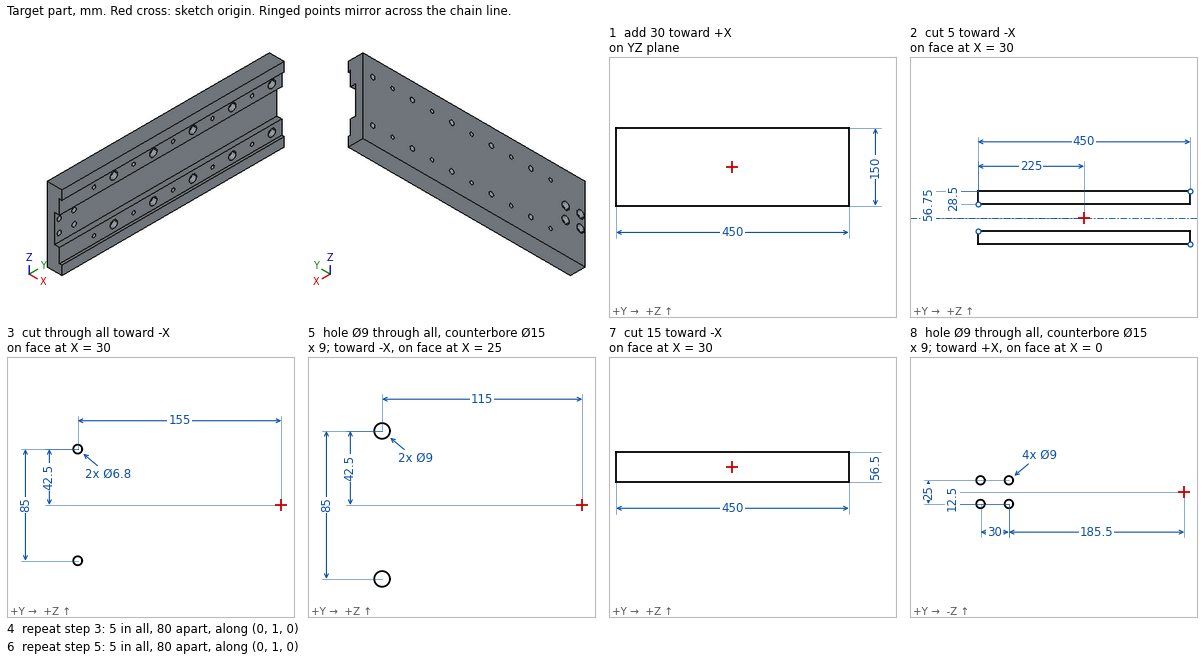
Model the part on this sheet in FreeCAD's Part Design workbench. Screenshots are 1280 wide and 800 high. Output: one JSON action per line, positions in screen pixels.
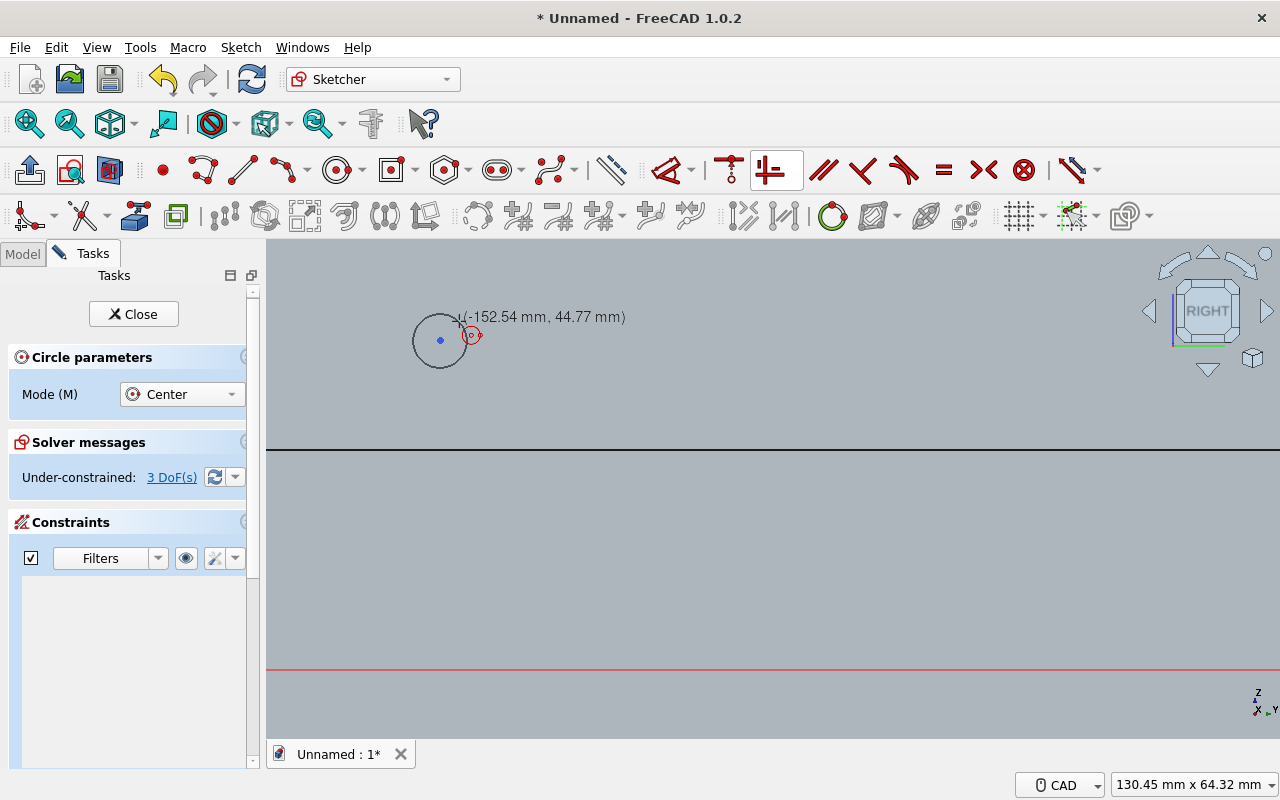
{"action": "scroll", "coordinate": [440, 341], "scroll_direction": "down", "scroll_amount": 4}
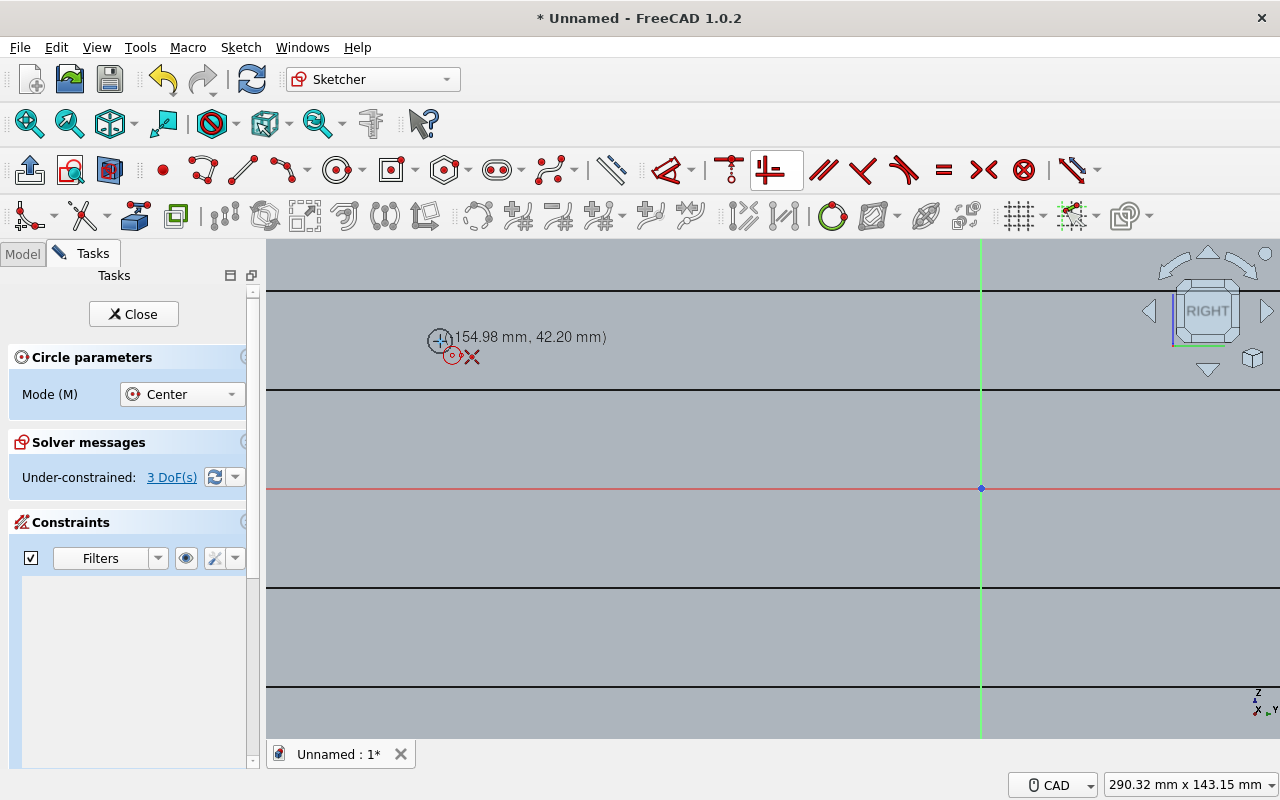
{"action": "scroll", "coordinate": [440, 637], "scroll_direction": "up", "scroll_amount": 4}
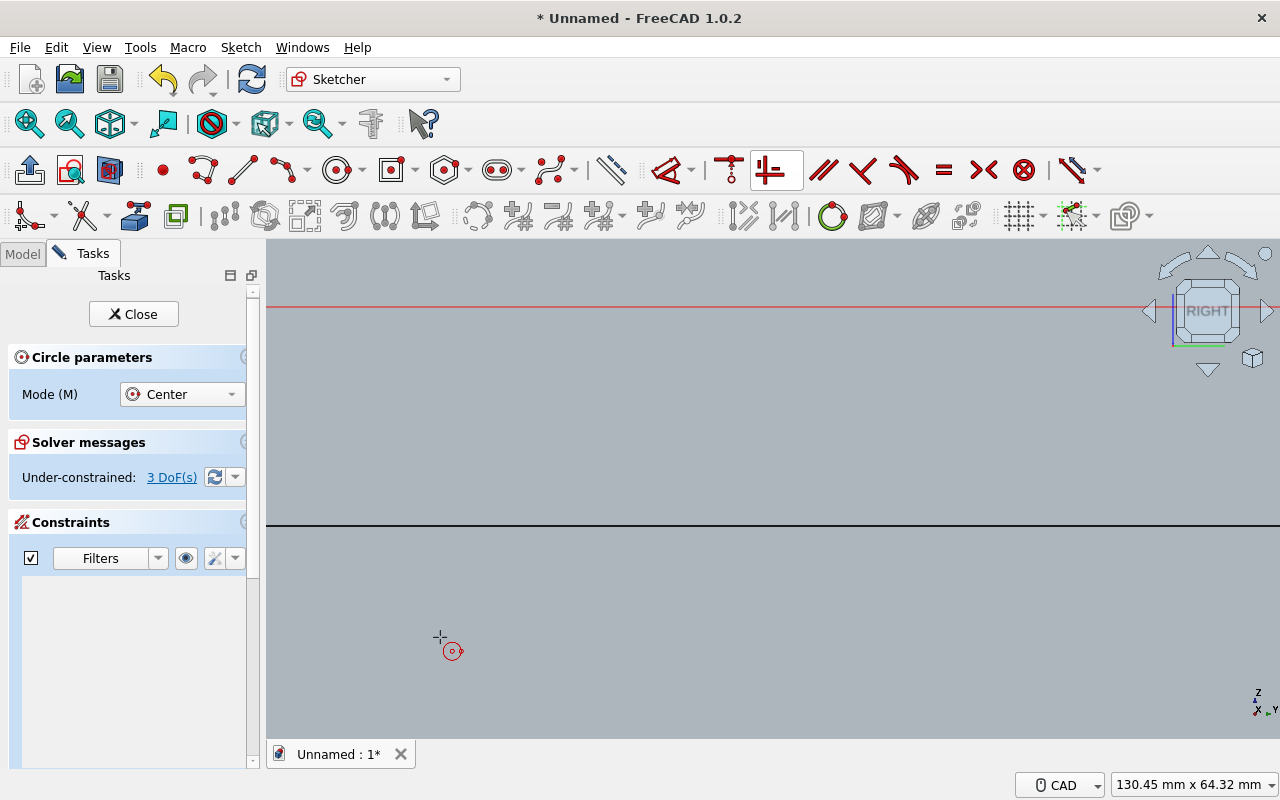
{"action": "left_click", "coordinate": [440, 637]}
{"action": "left_click", "coordinate": [459, 618]}
{"action": "key", "text": "Escape"}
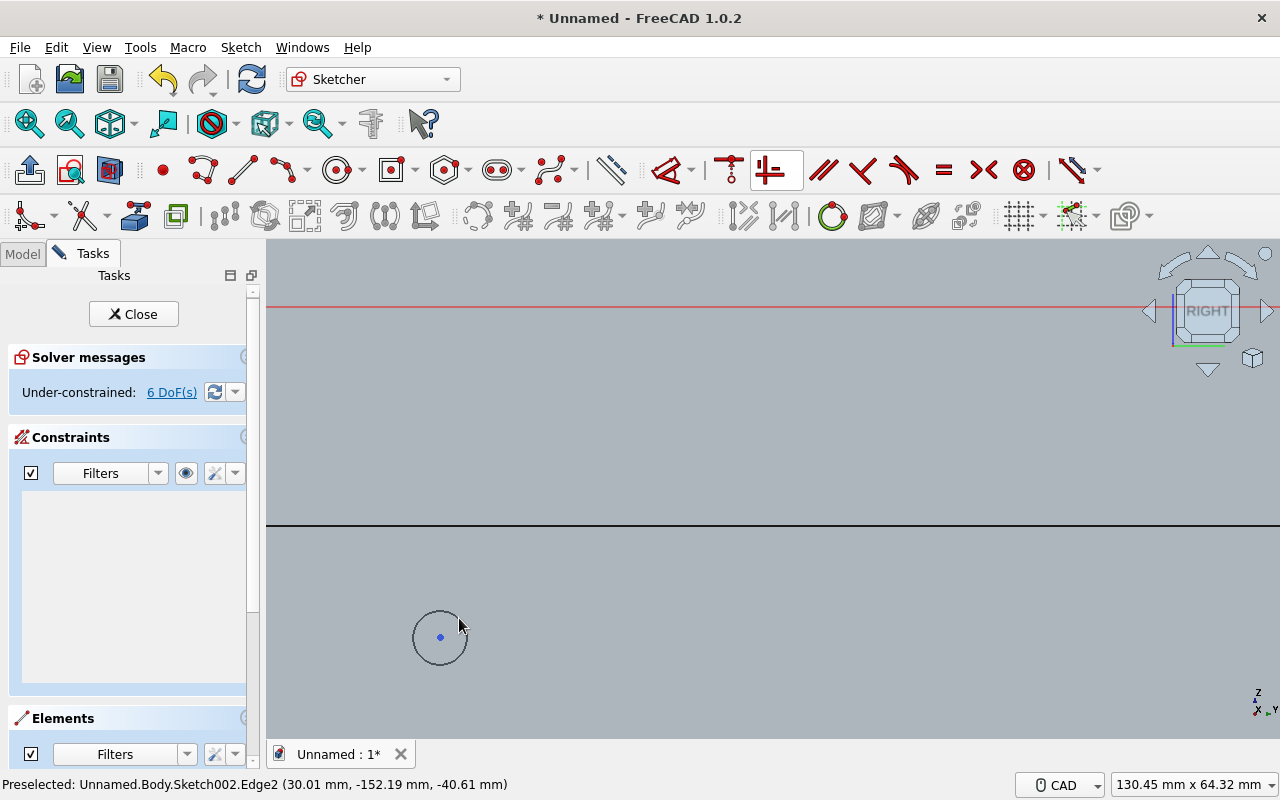
{"action": "scroll", "coordinate": [440, 638], "scroll_direction": "down", "scroll_amount": 4}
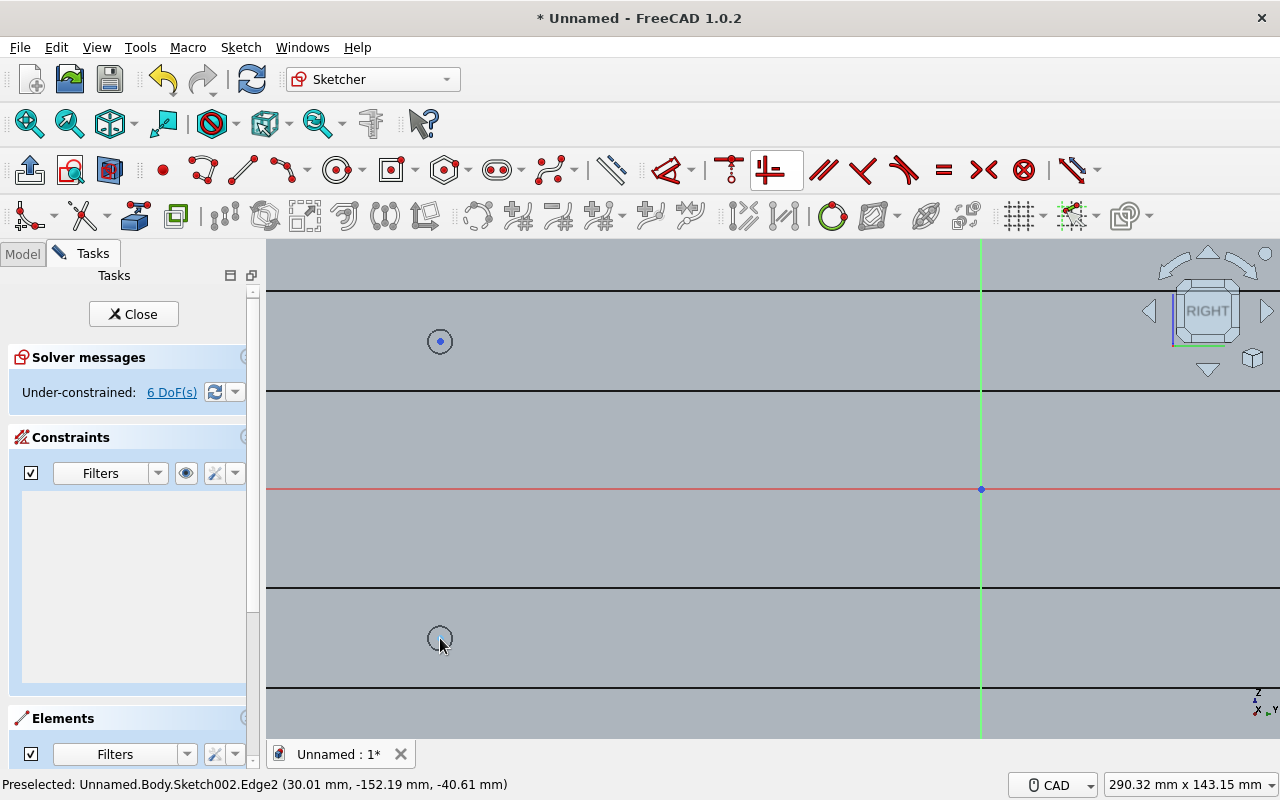
{"action": "left_click", "coordinate": [449, 333]}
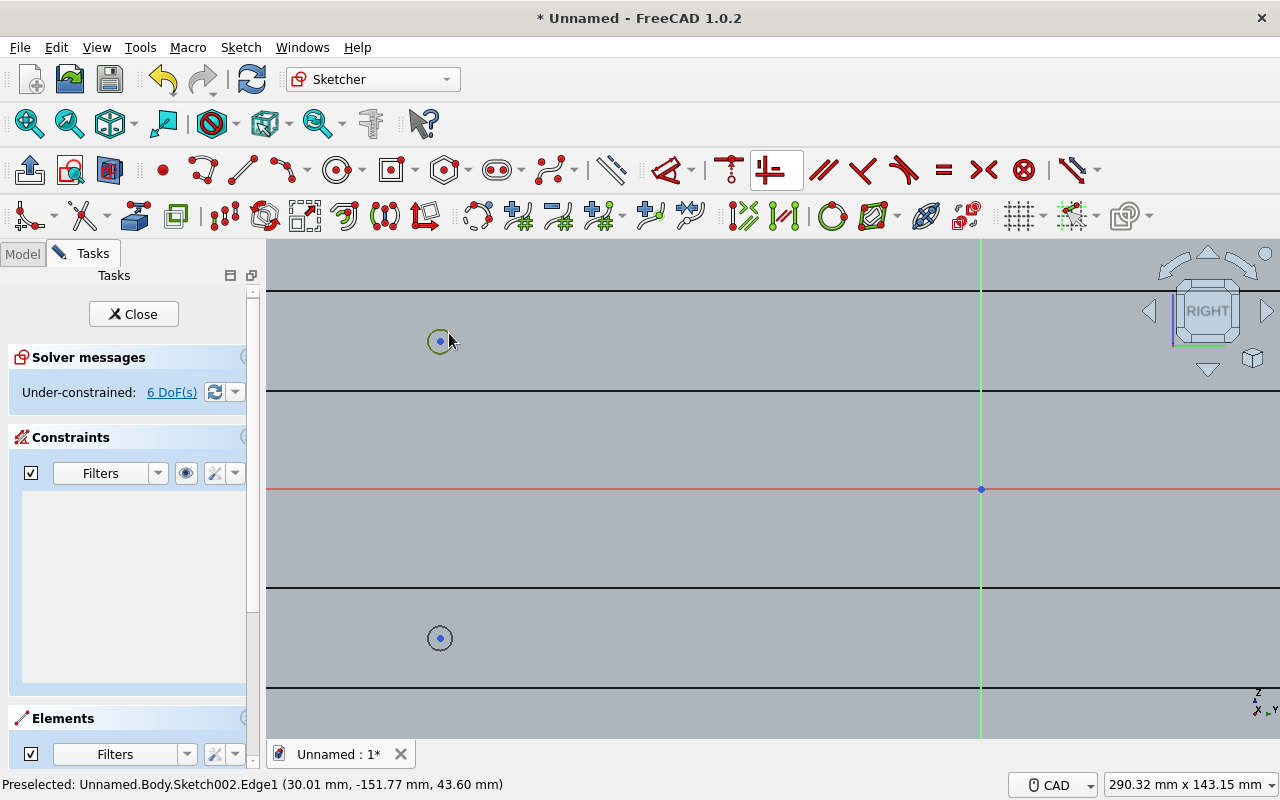
{"action": "left_click", "coordinate": [449, 630]}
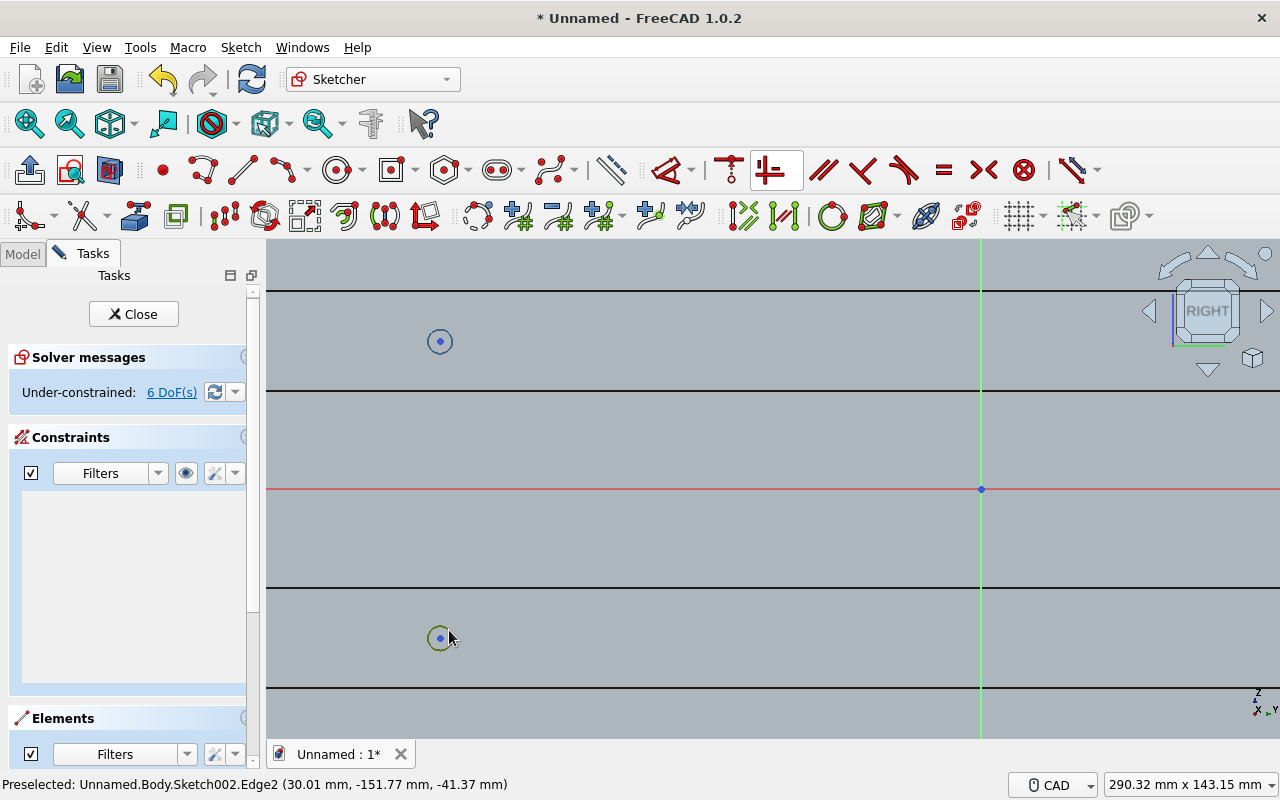
{"action": "key", "text": "e"}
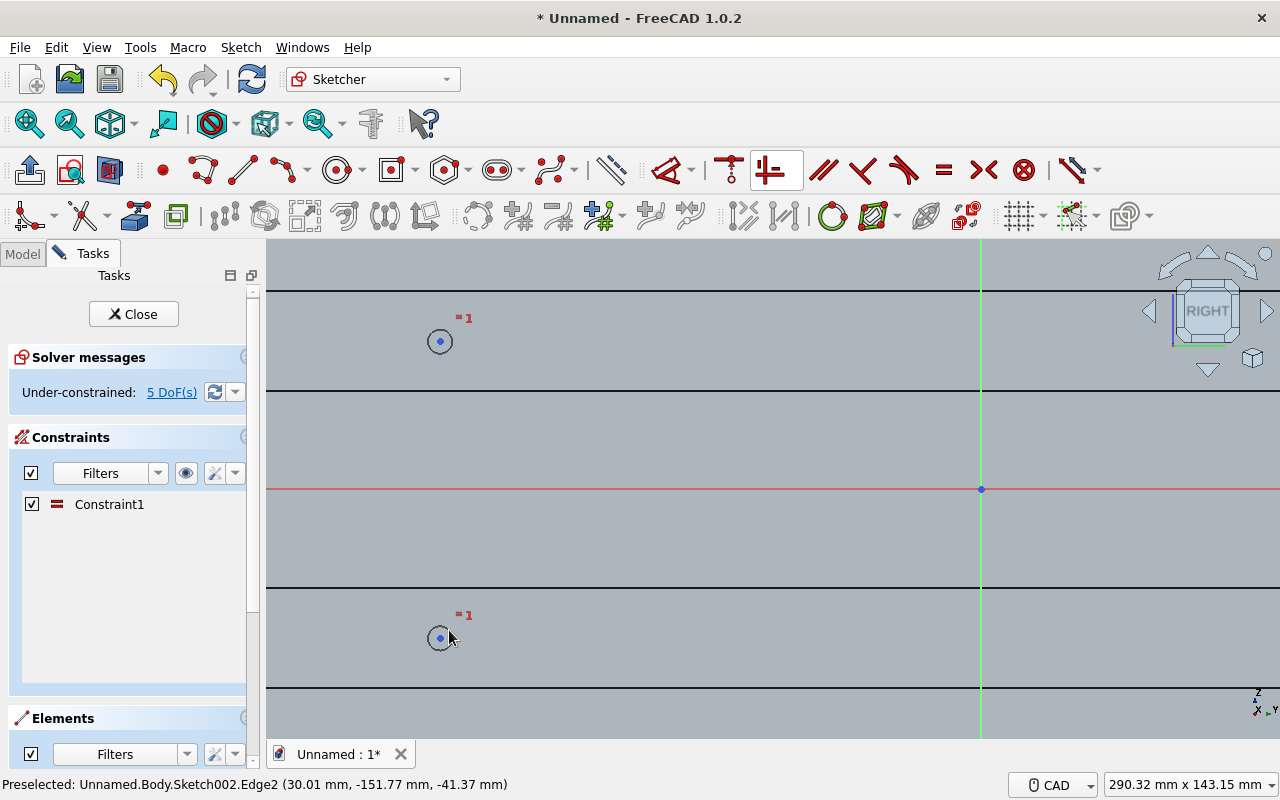
{"action": "left_click", "coordinate": [440, 342]}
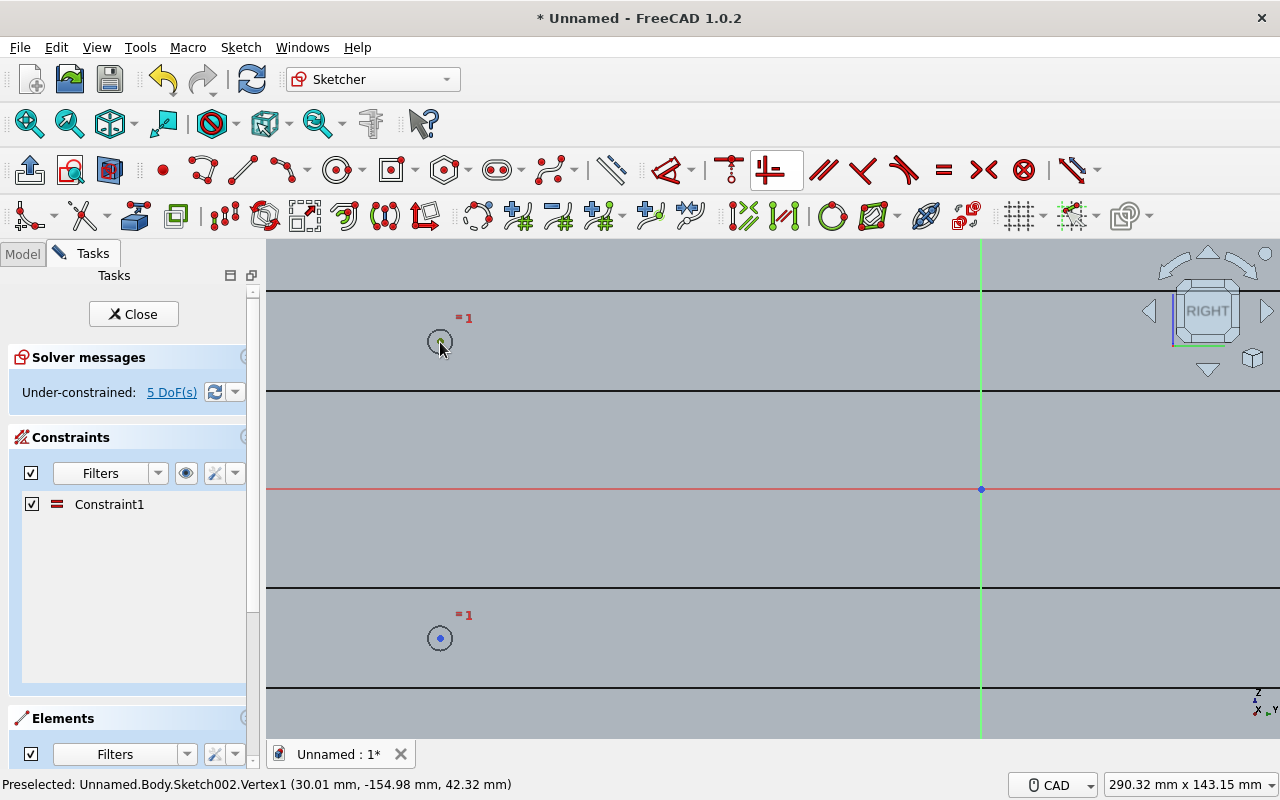
{"action": "left_click", "coordinate": [440, 638]}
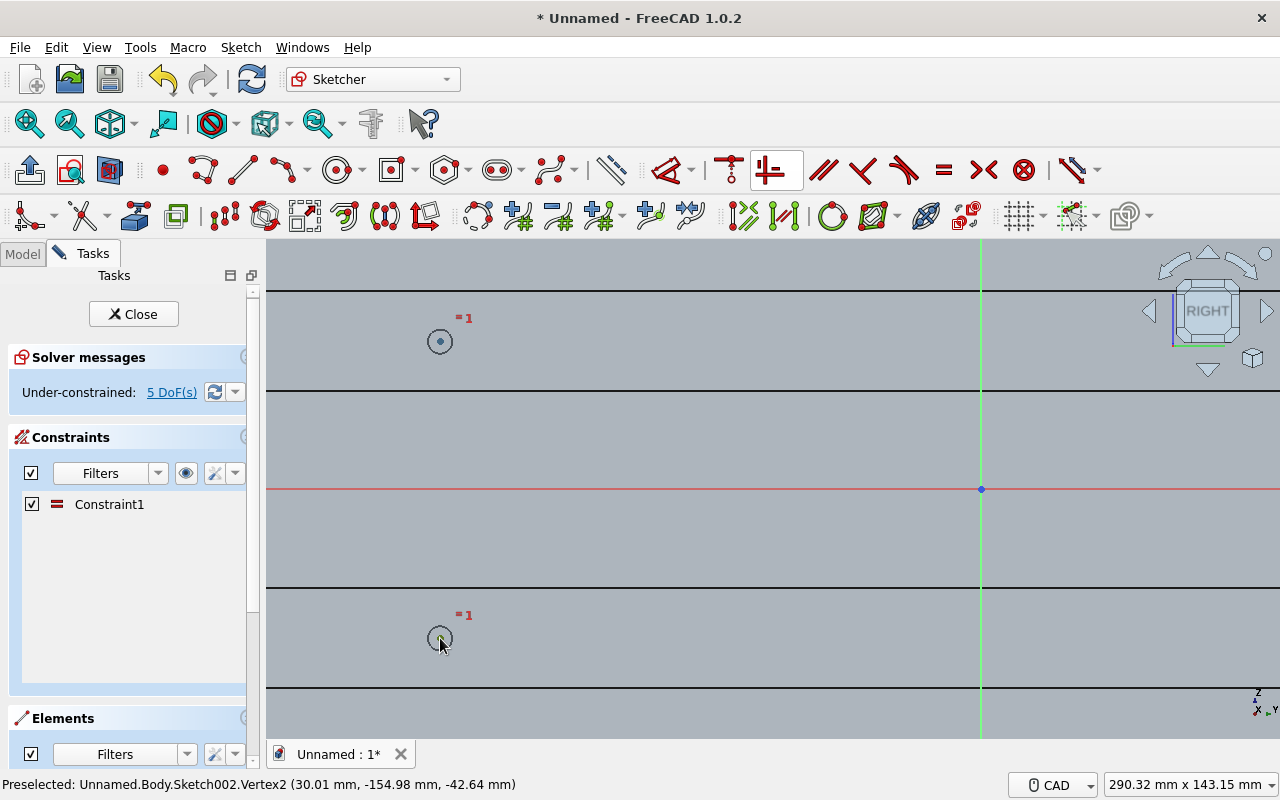
{"action": "key", "text": "v"}